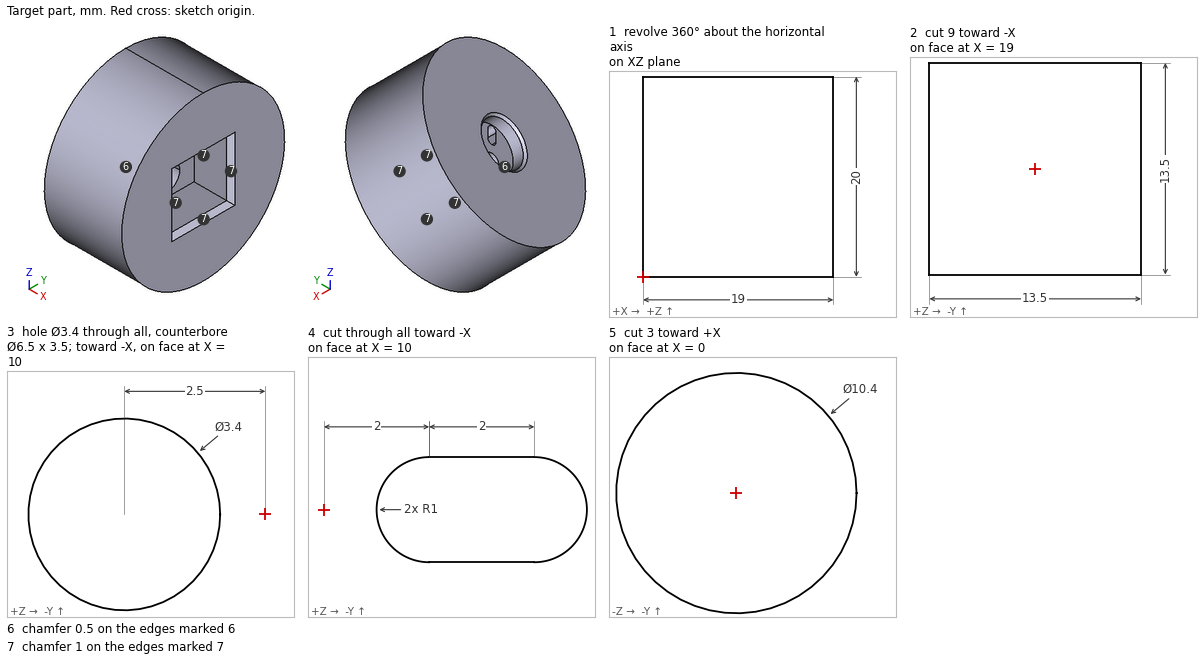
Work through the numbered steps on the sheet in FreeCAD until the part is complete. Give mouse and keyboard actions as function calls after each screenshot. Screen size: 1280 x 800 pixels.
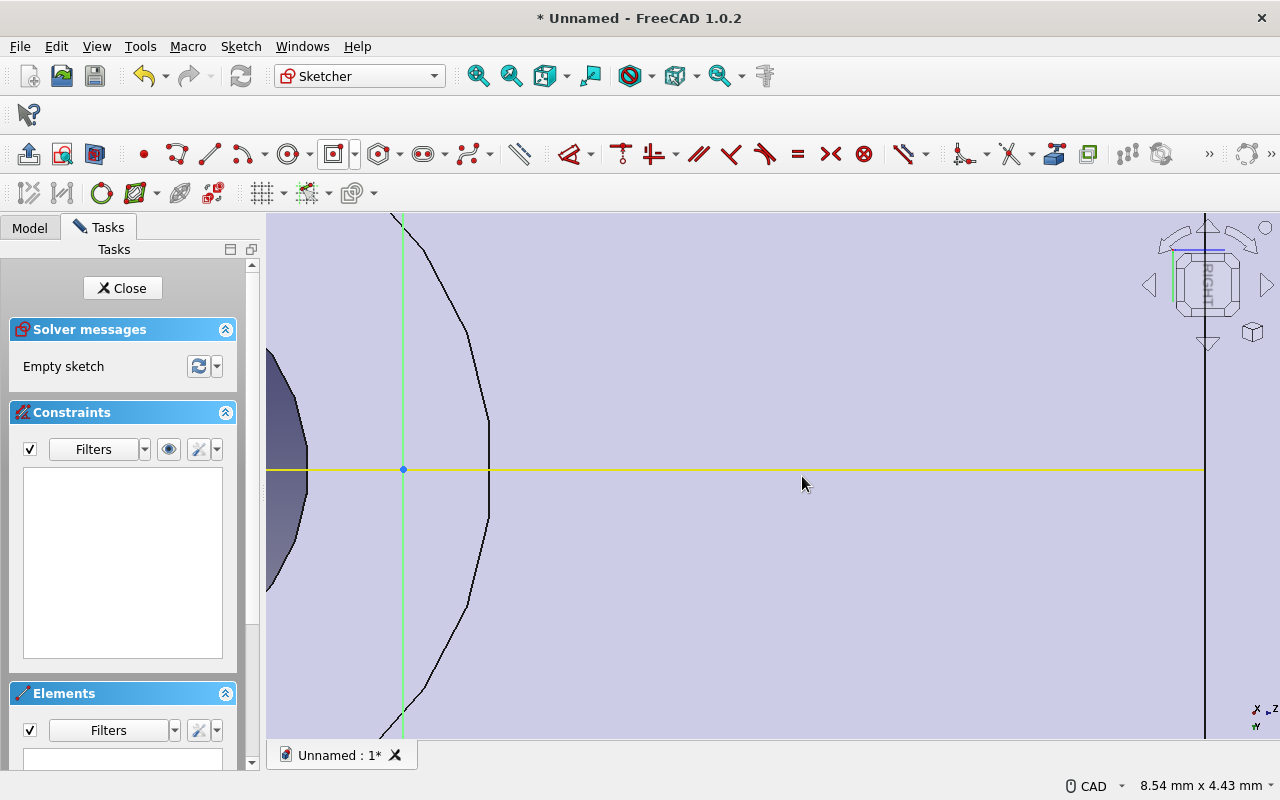
click(422, 154)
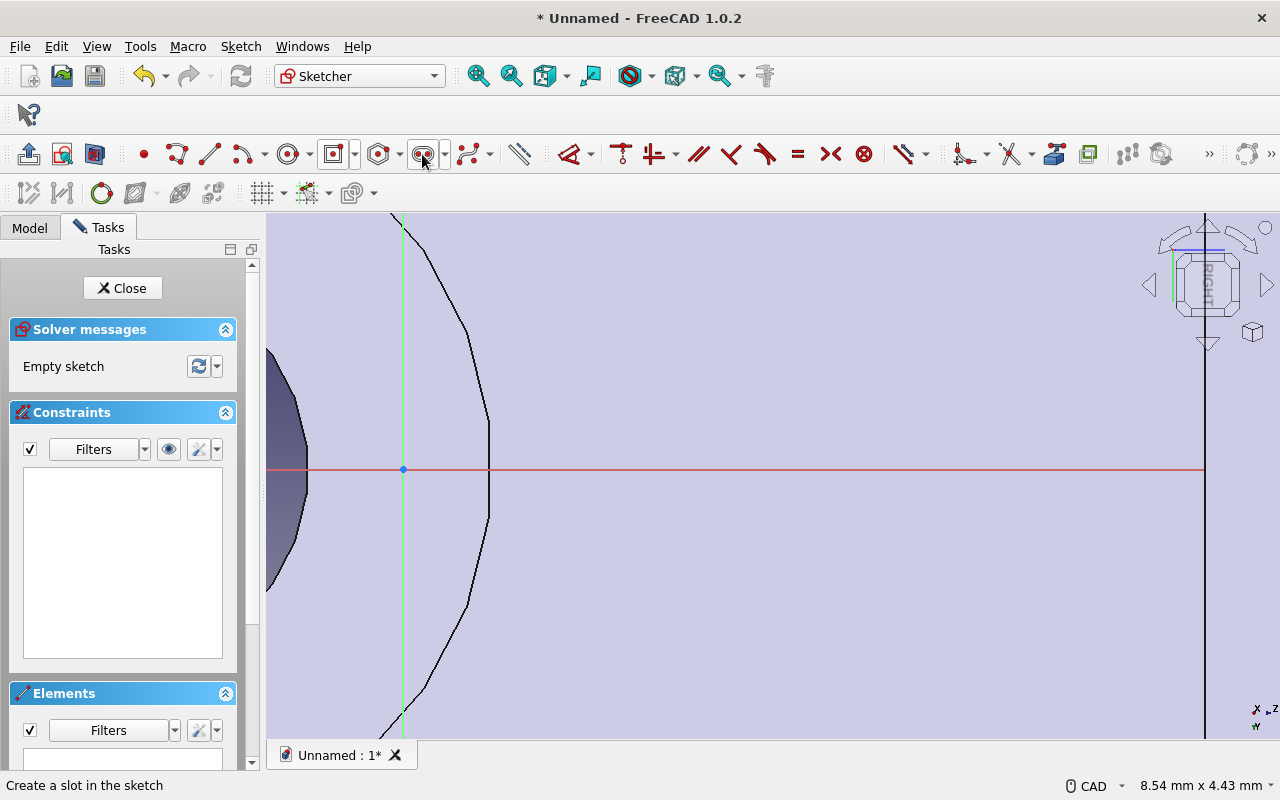
click(641, 470)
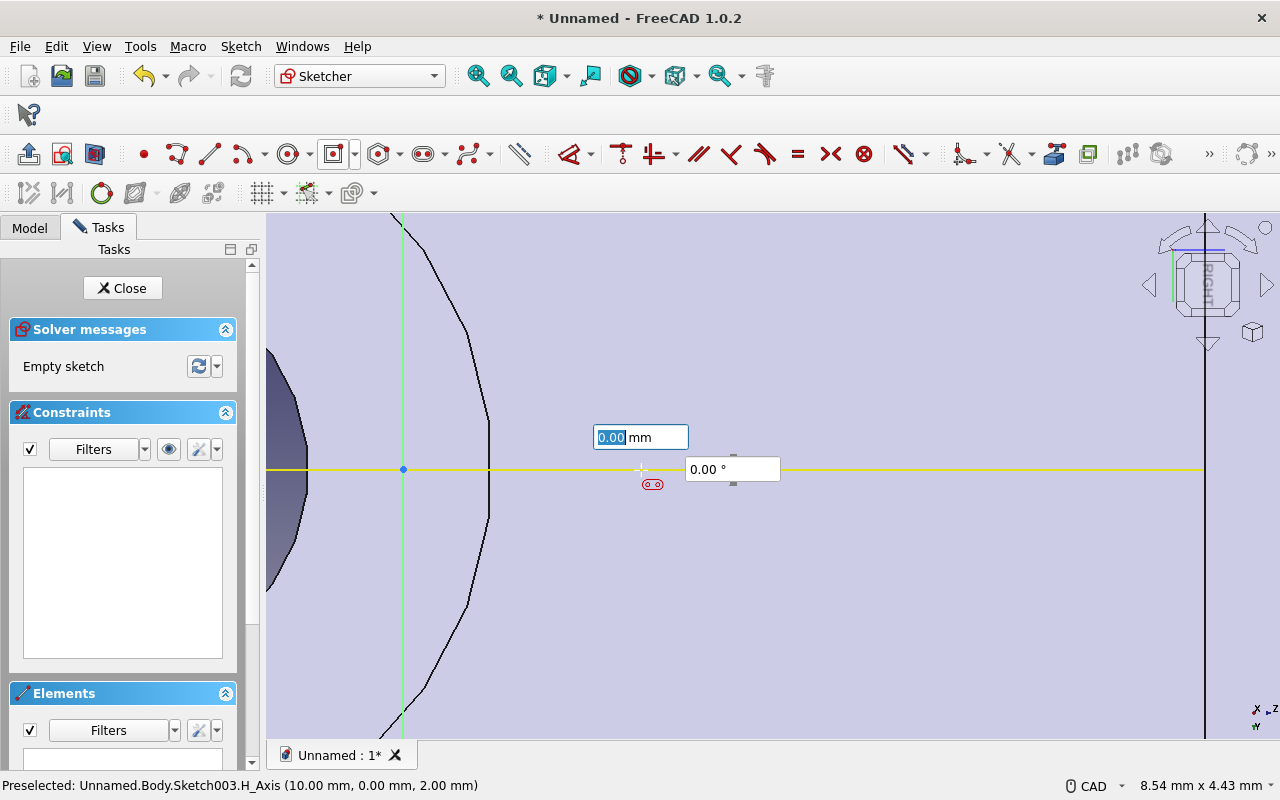
click(878, 461)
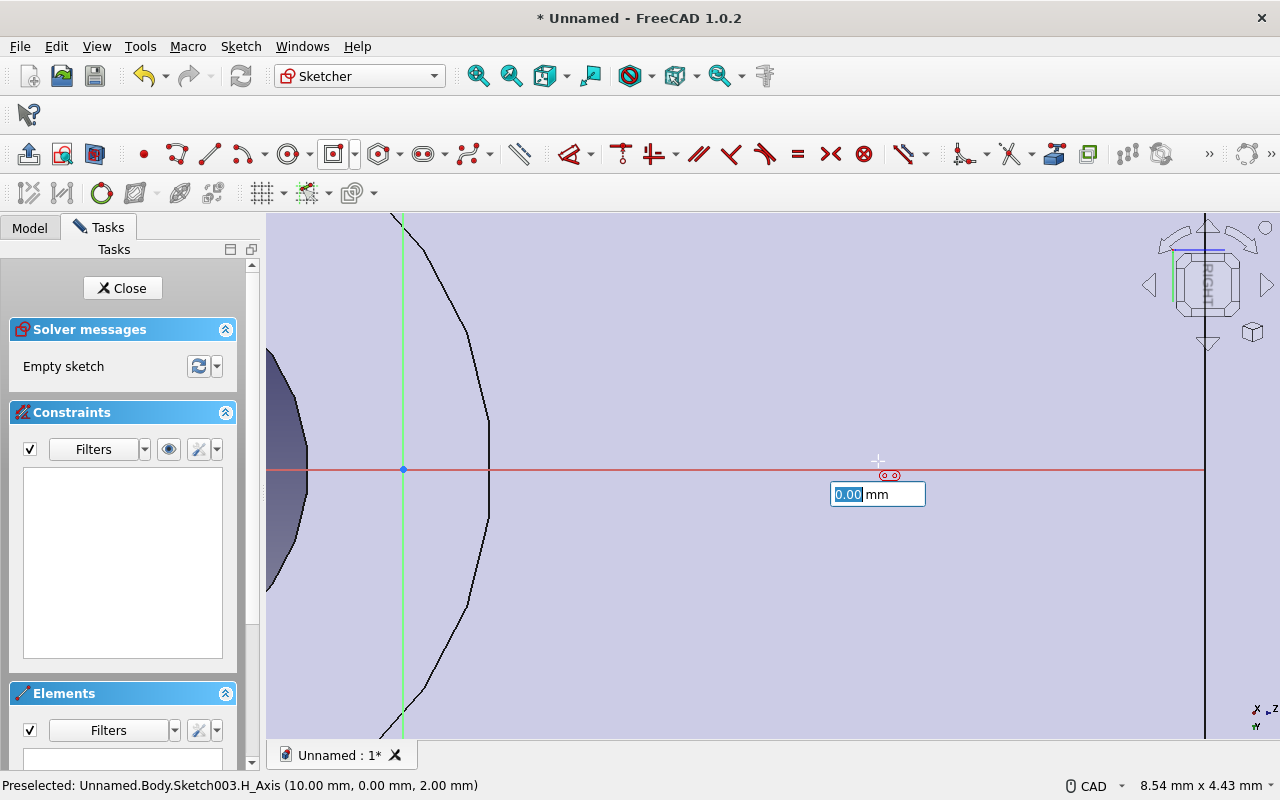
click(759, 351)
key(Escape)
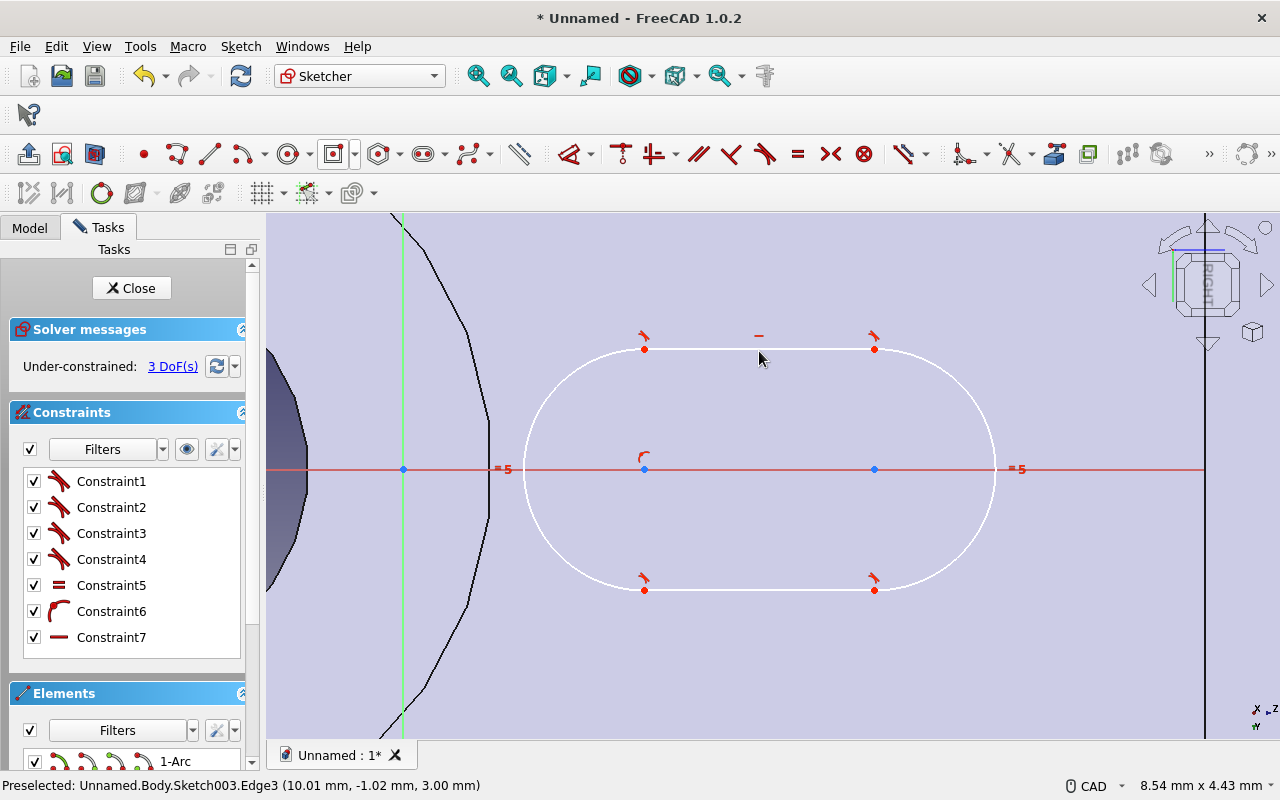
click(568, 154)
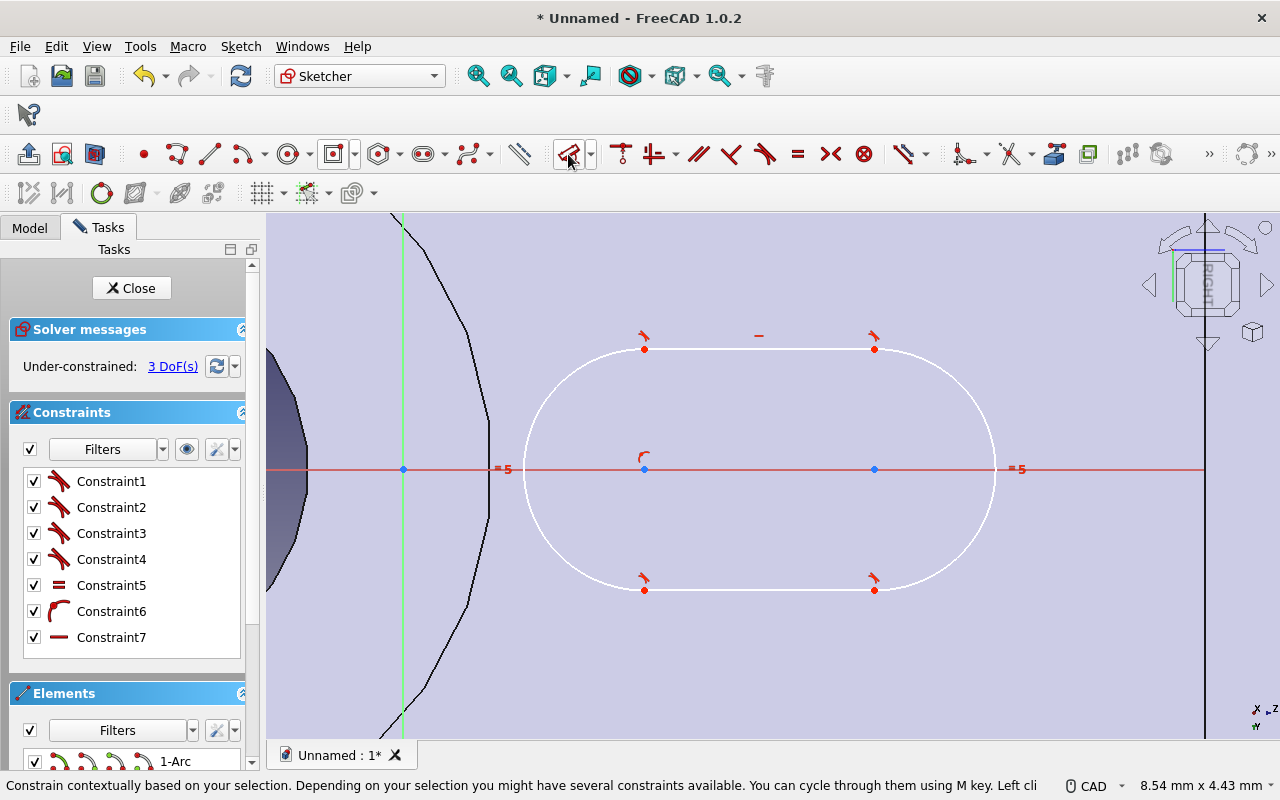
click(547, 399)
click(521, 380)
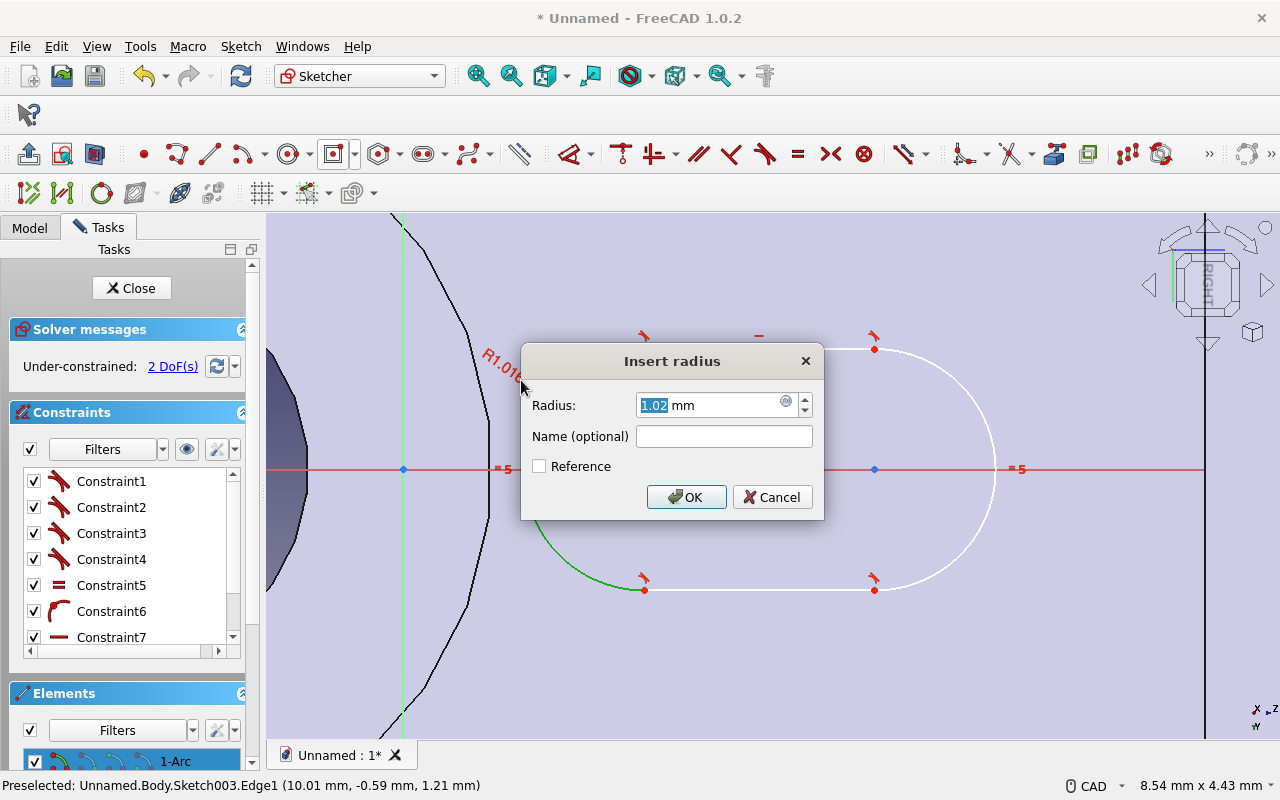
text(1)
key(Return)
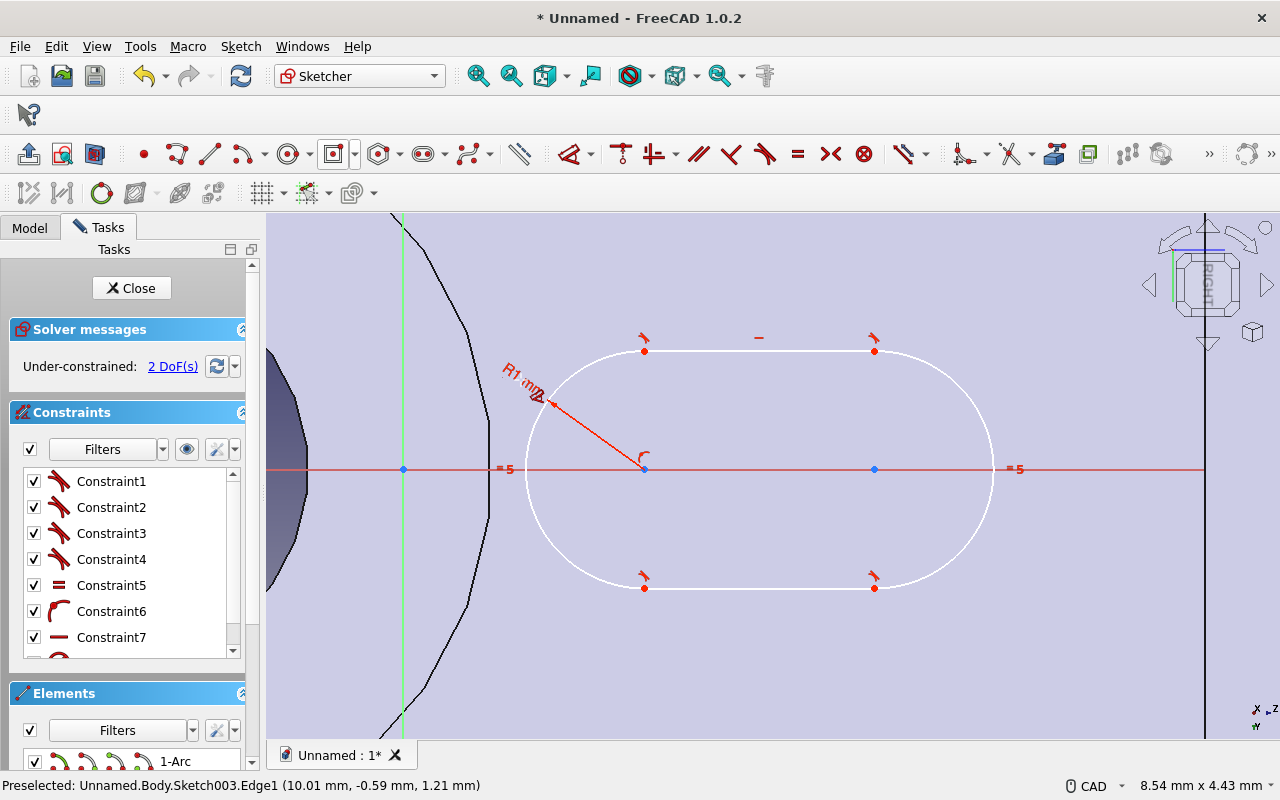
click(714, 351)
click(760, 317)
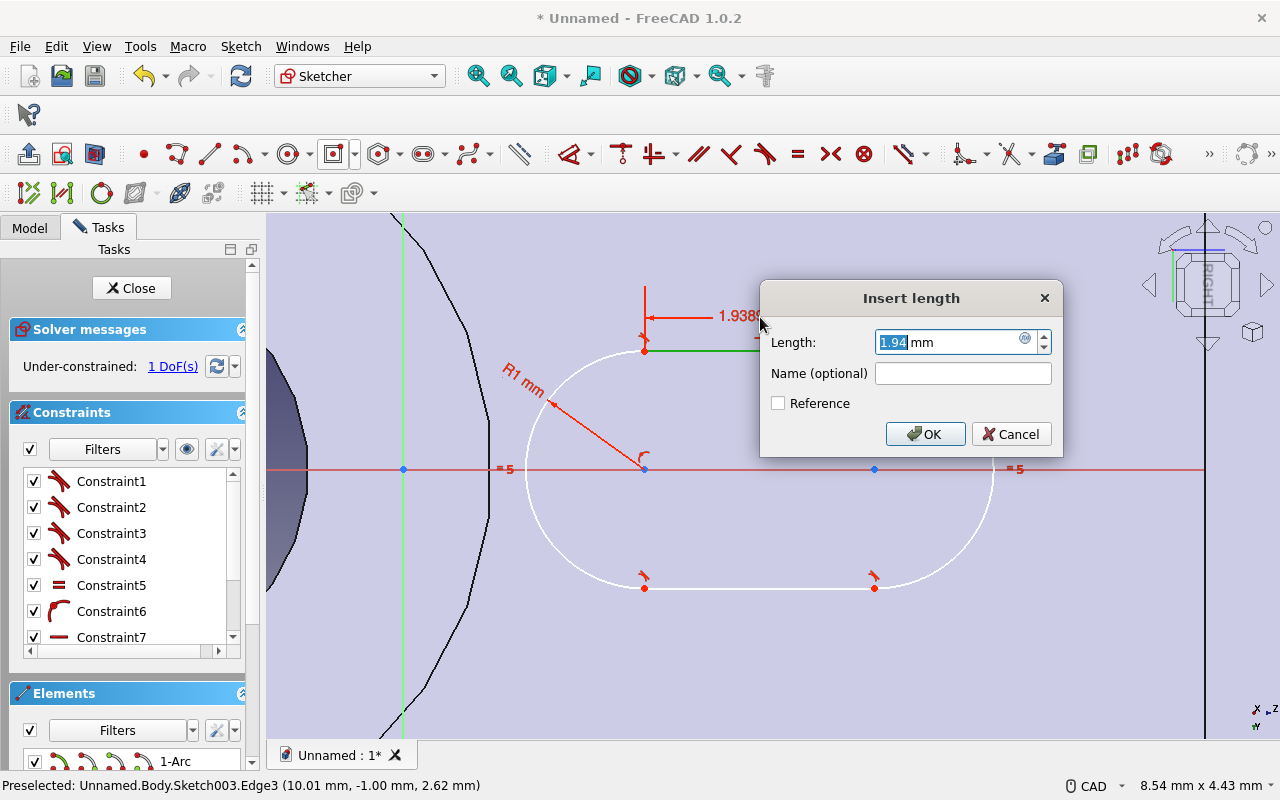
text(2)
key(Return)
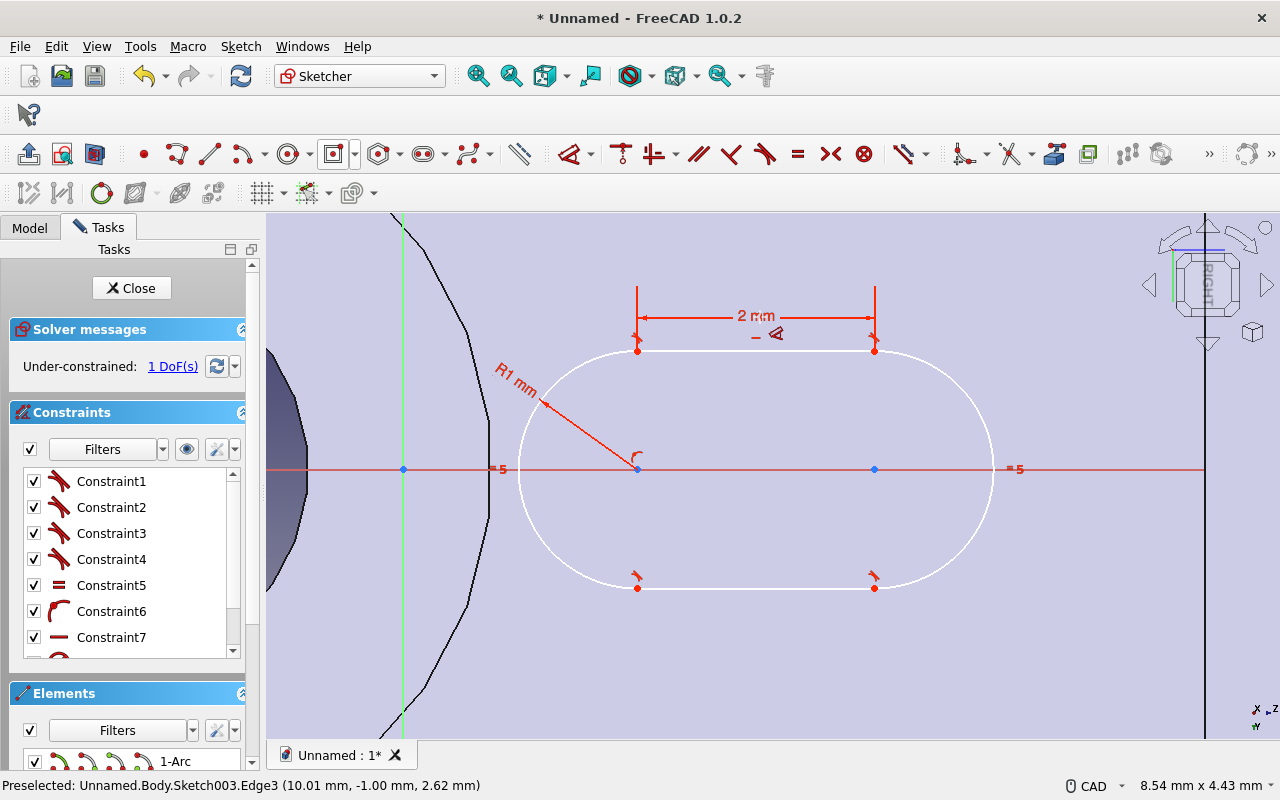
click(637, 351)
click(520, 317)